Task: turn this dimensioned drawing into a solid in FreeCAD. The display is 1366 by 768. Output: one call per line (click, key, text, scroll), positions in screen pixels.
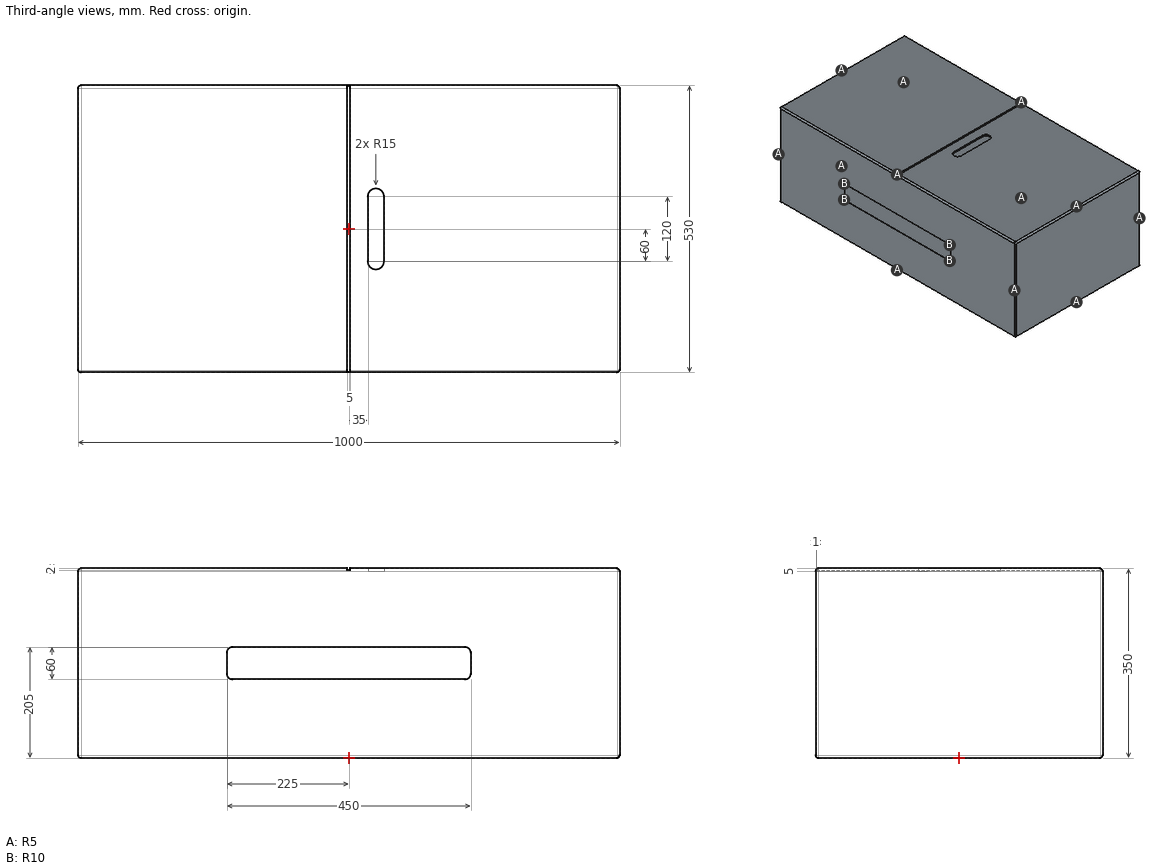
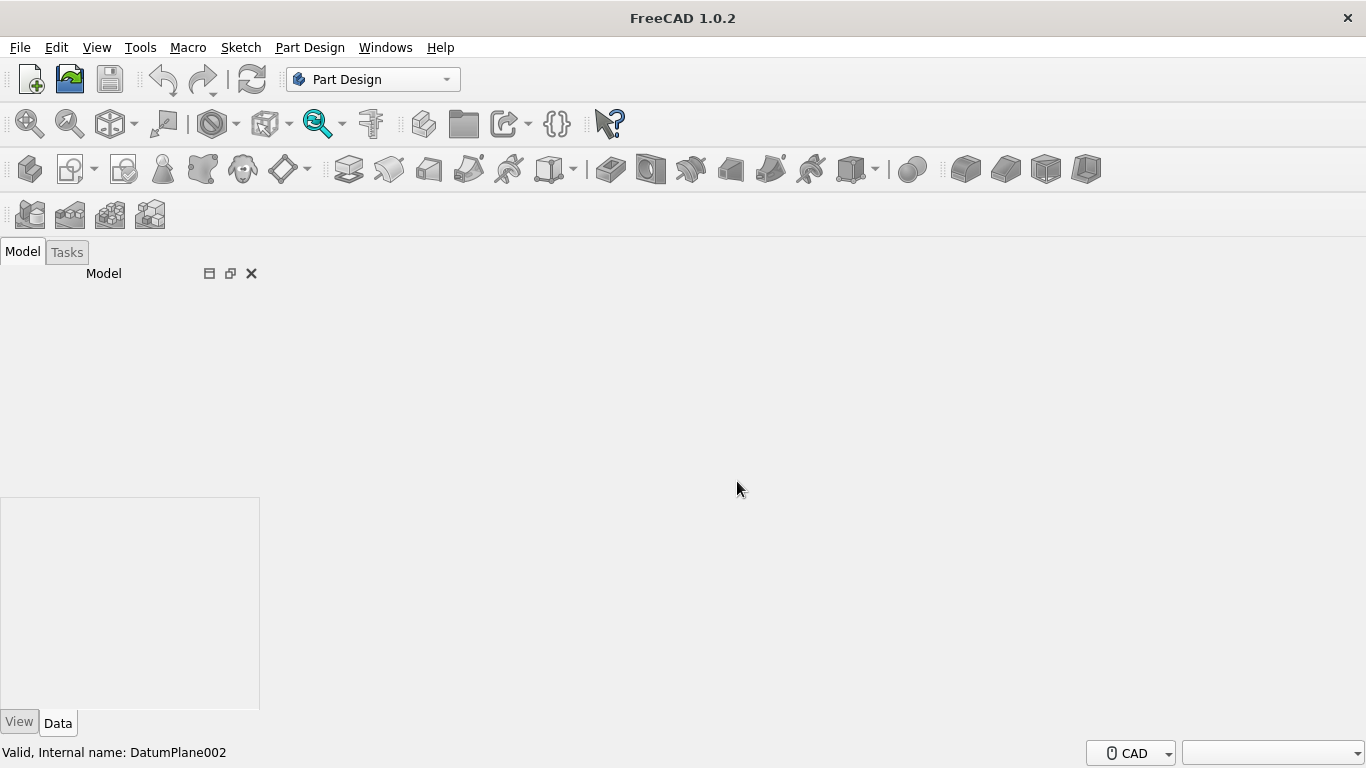
click(30, 80)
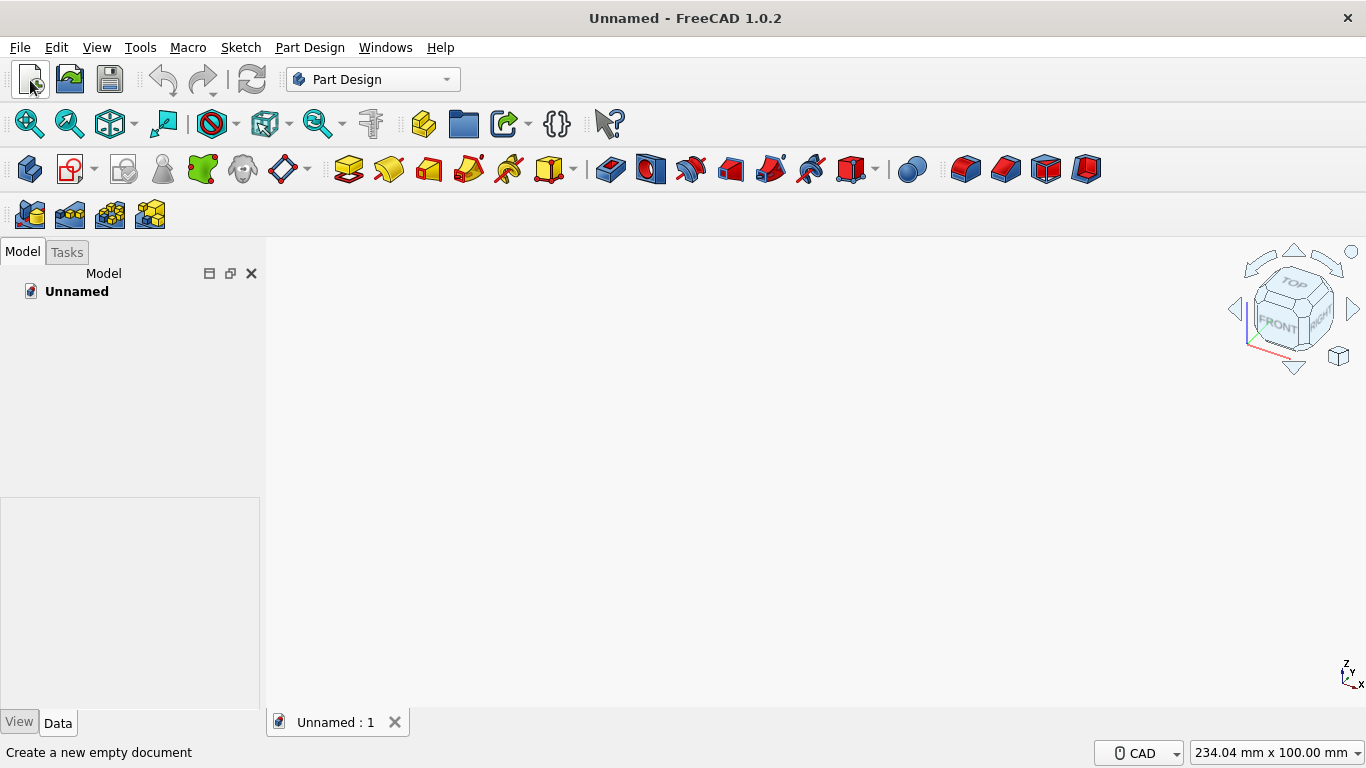
click(70, 170)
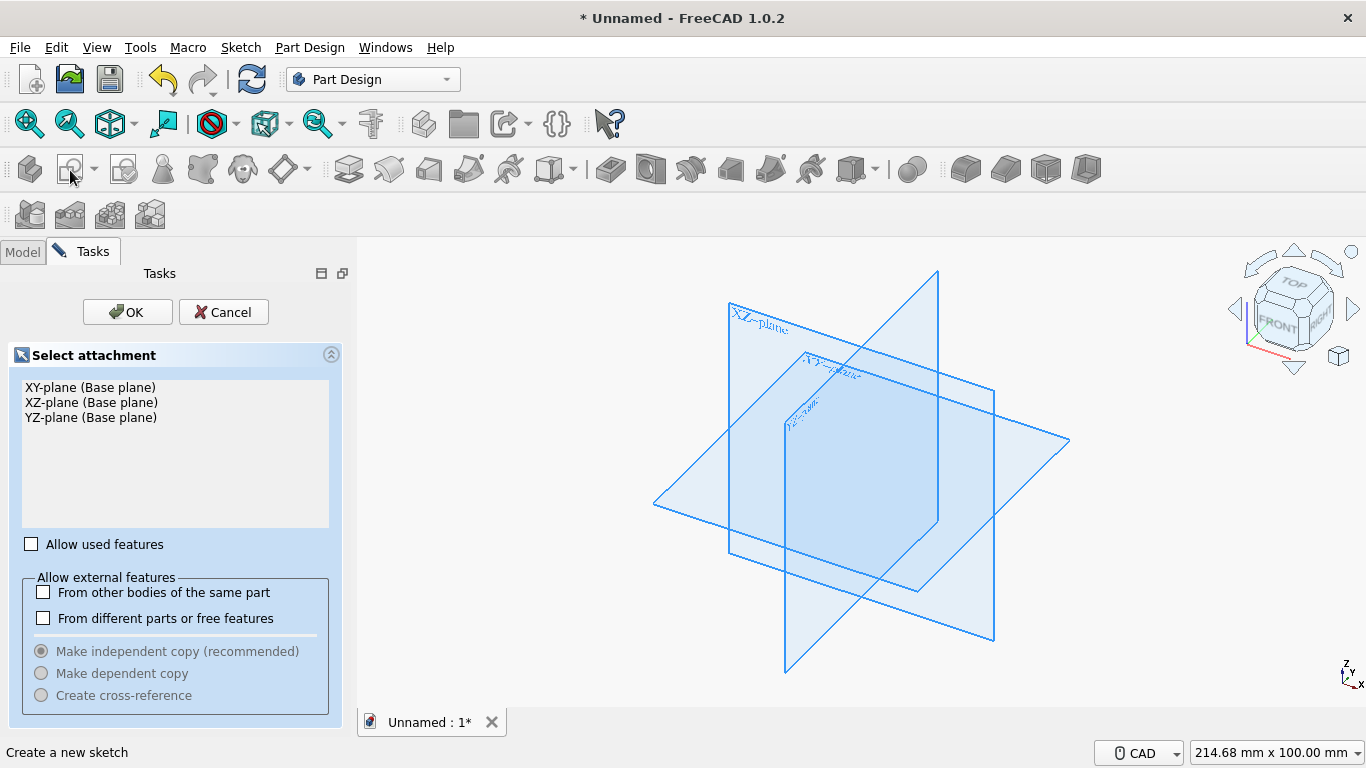
click(82, 388)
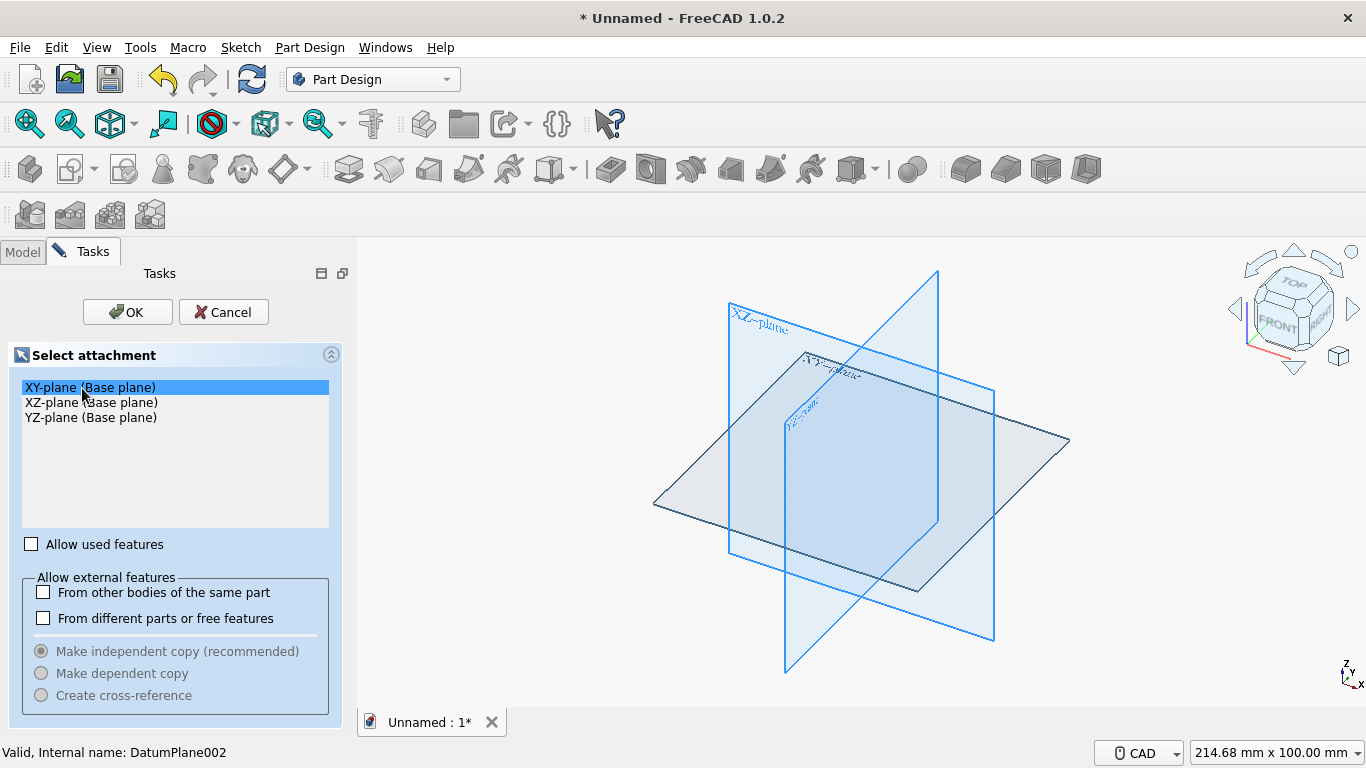
click(128, 312)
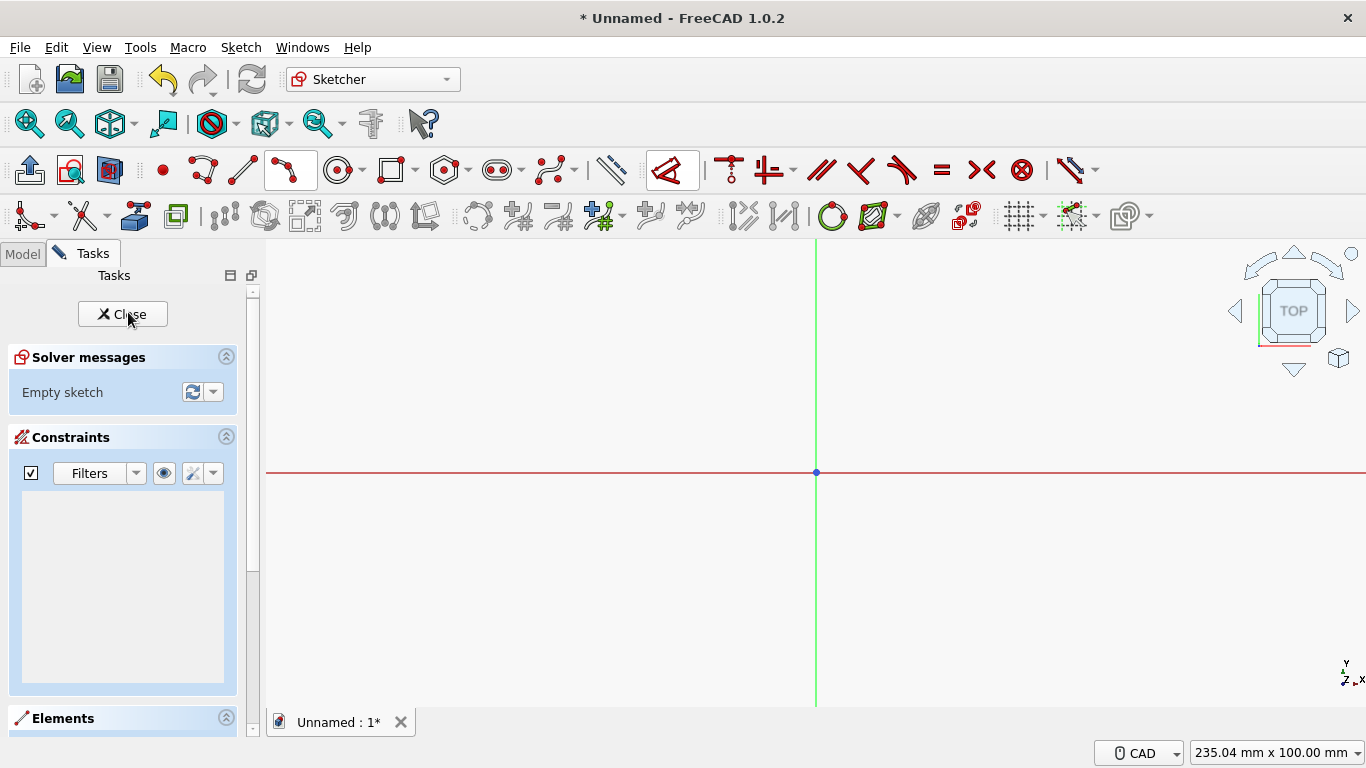
scroll(739, 473, down, 11)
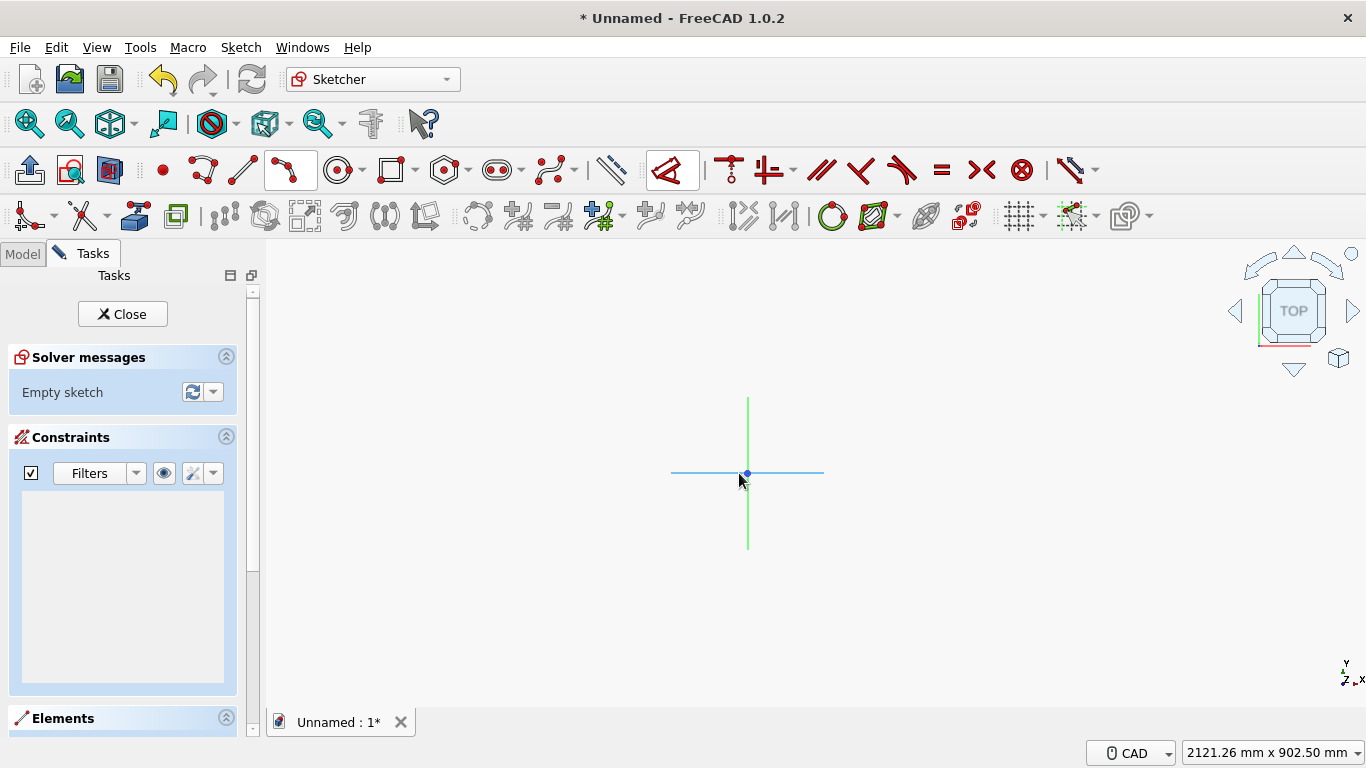
click(418, 170)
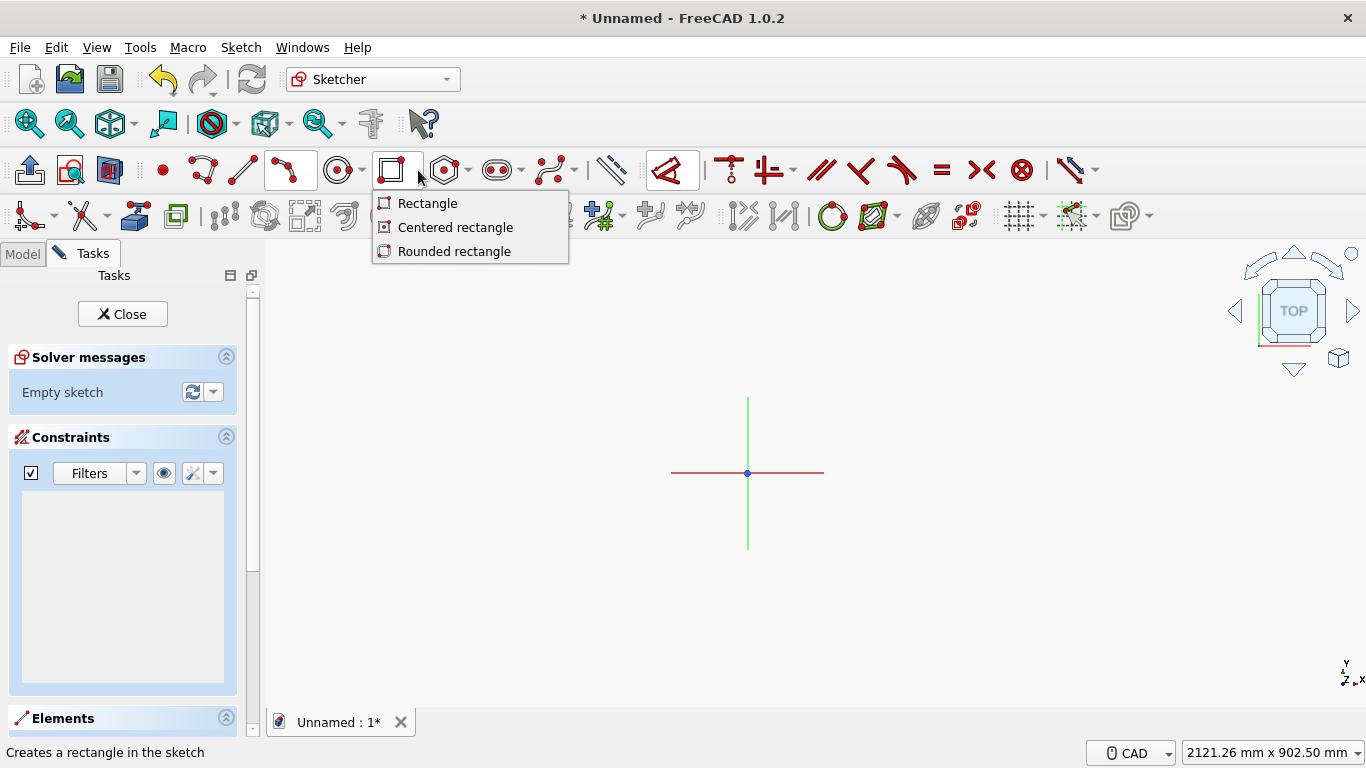
click(470, 227)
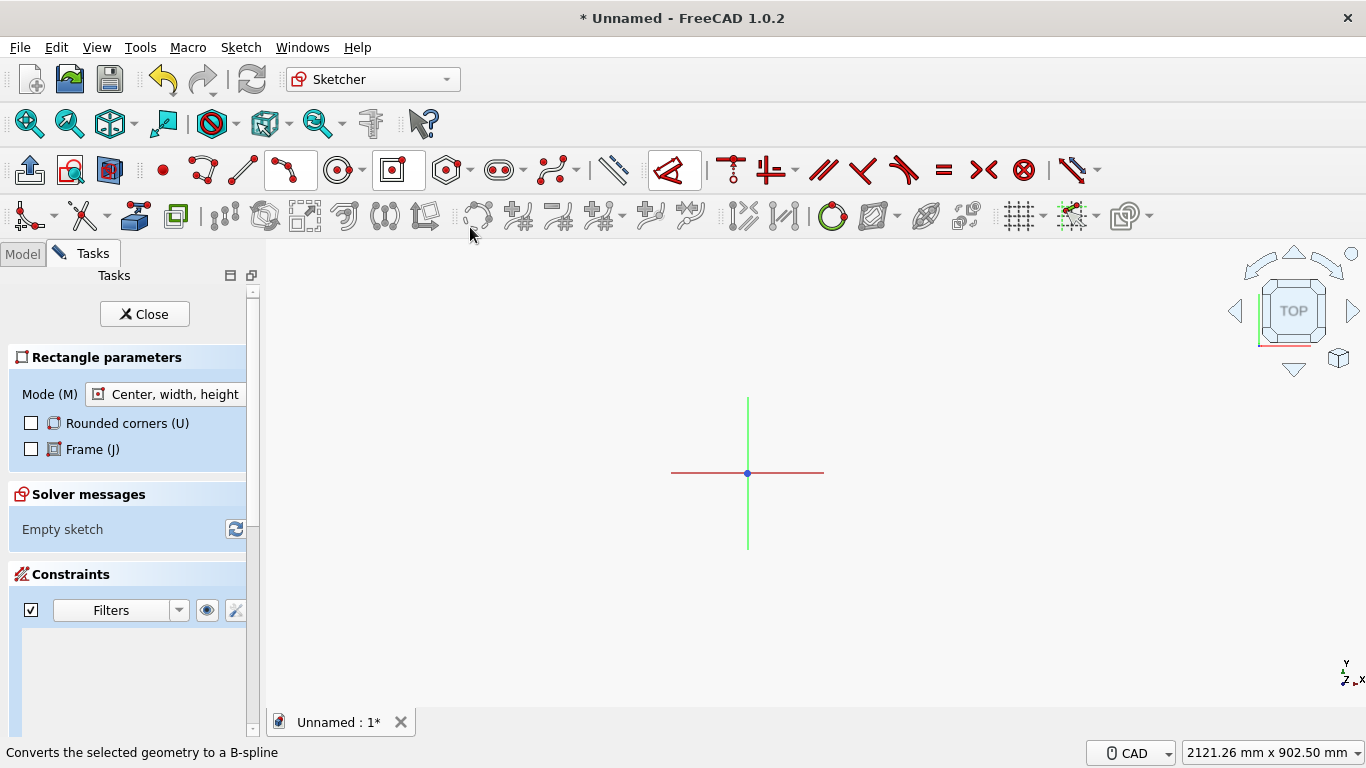
click(748, 473)
click(1007, 336)
key(Escape)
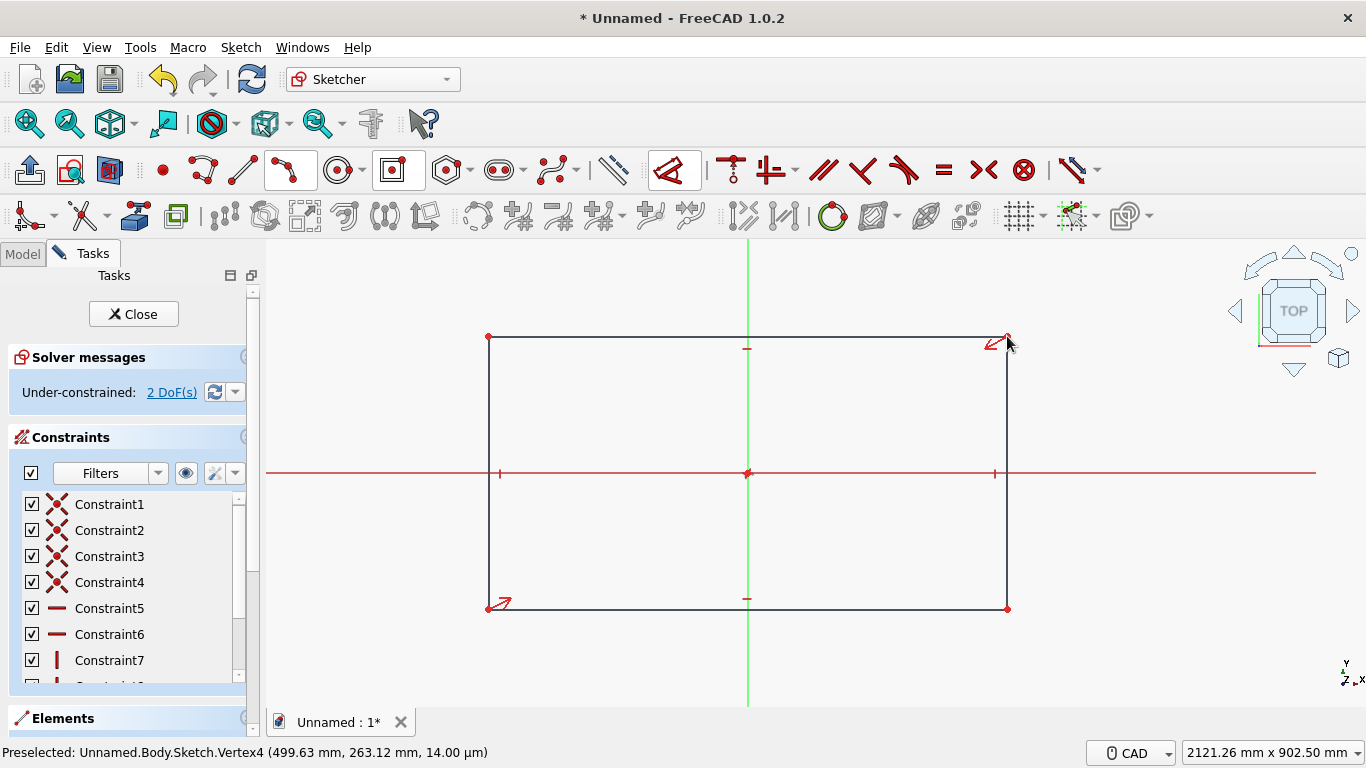
click(668, 170)